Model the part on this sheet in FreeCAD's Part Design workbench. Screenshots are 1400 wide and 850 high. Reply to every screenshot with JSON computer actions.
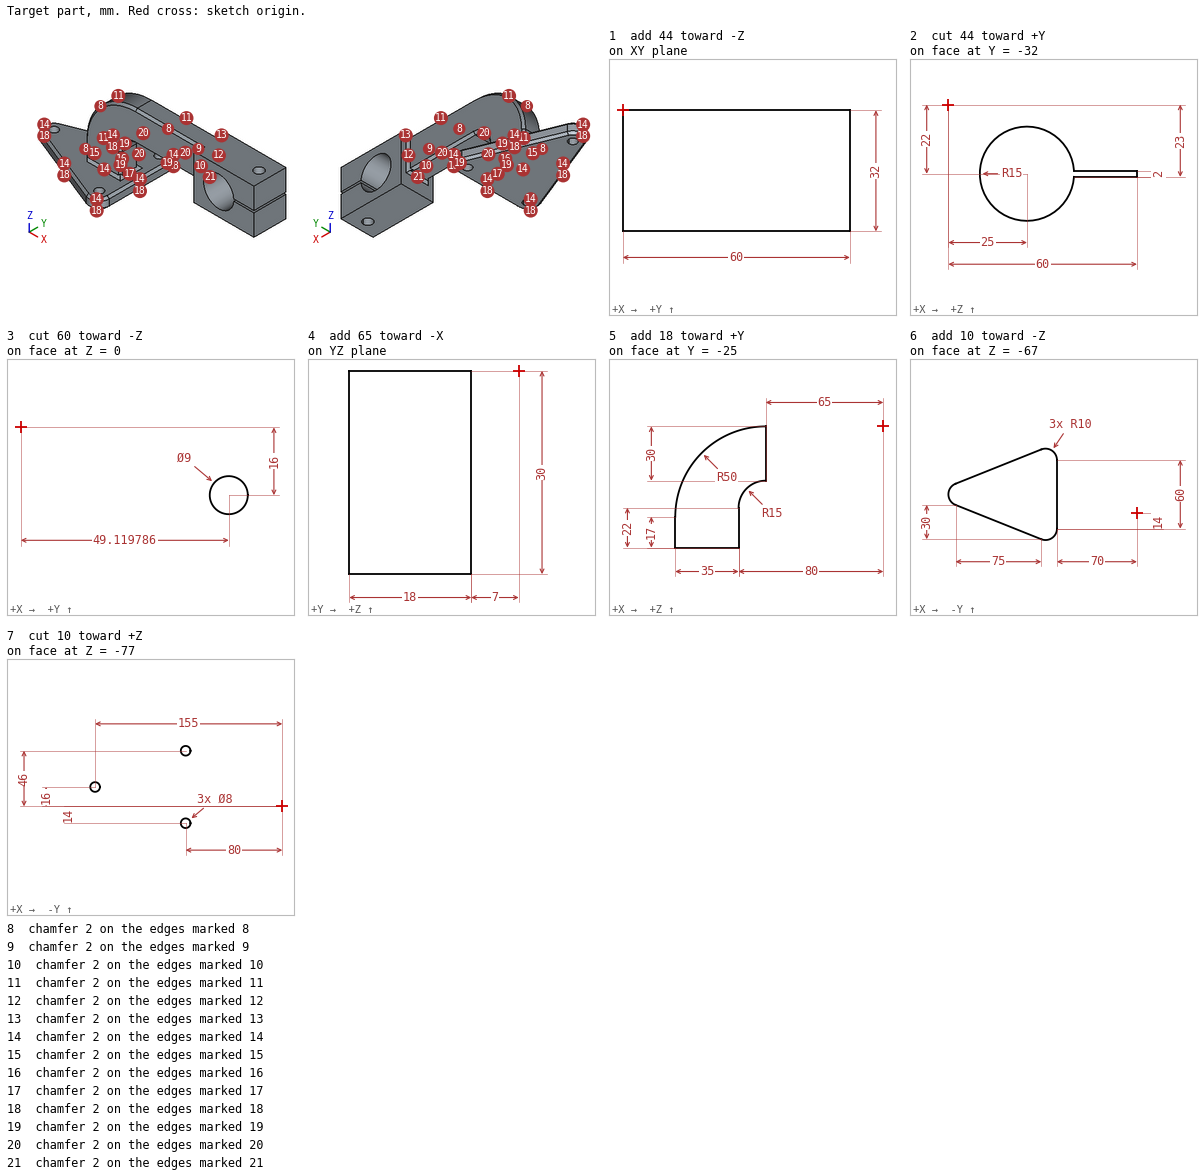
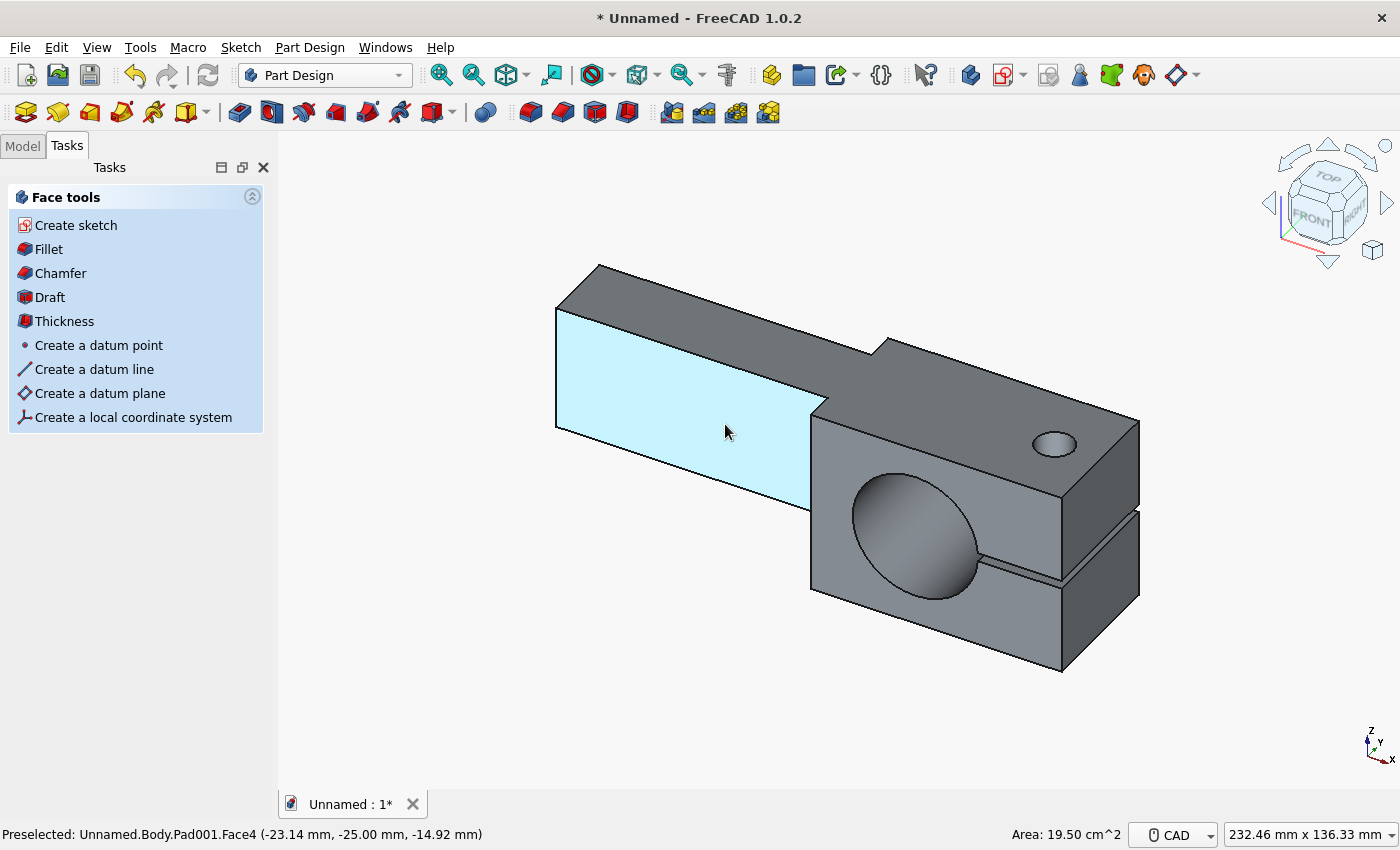
{"action": "left_click", "coordinate": [1004, 76]}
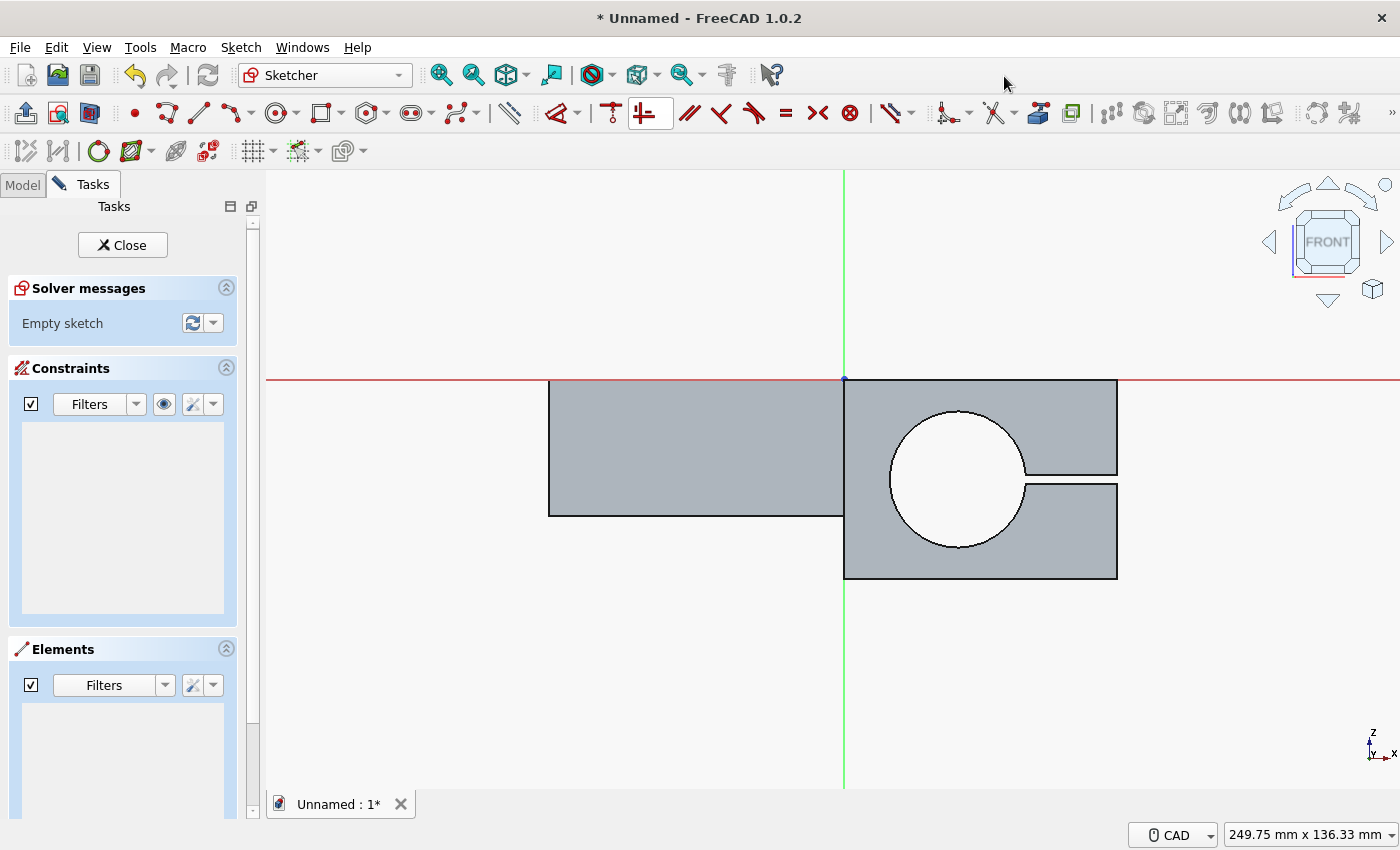
{"action": "left_click", "coordinate": [200, 114]}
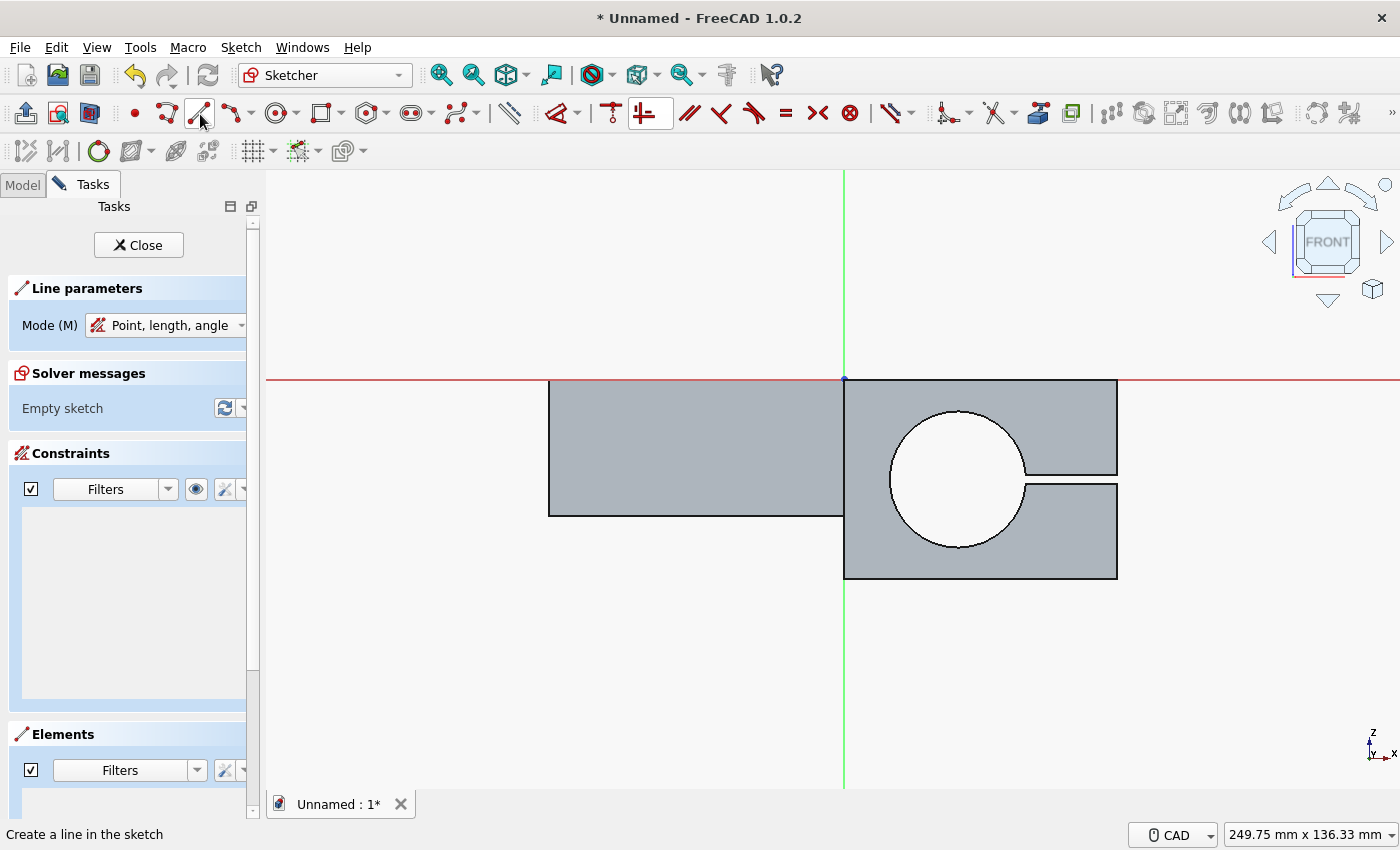
{"action": "left_click", "coordinate": [549, 516]}
{"action": "left_click", "coordinate": [549, 380]}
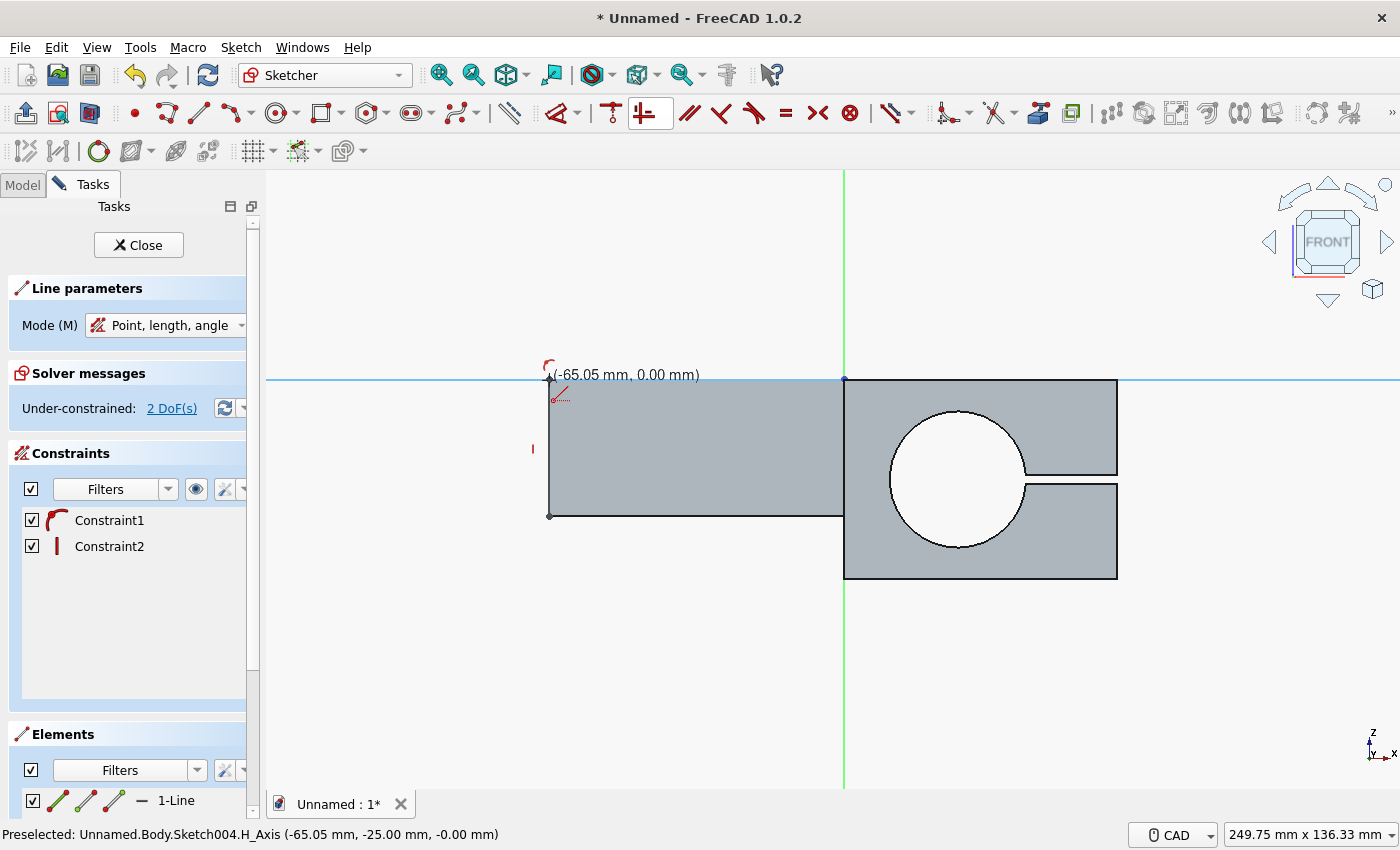
{"action": "left_click", "coordinate": [168, 114]}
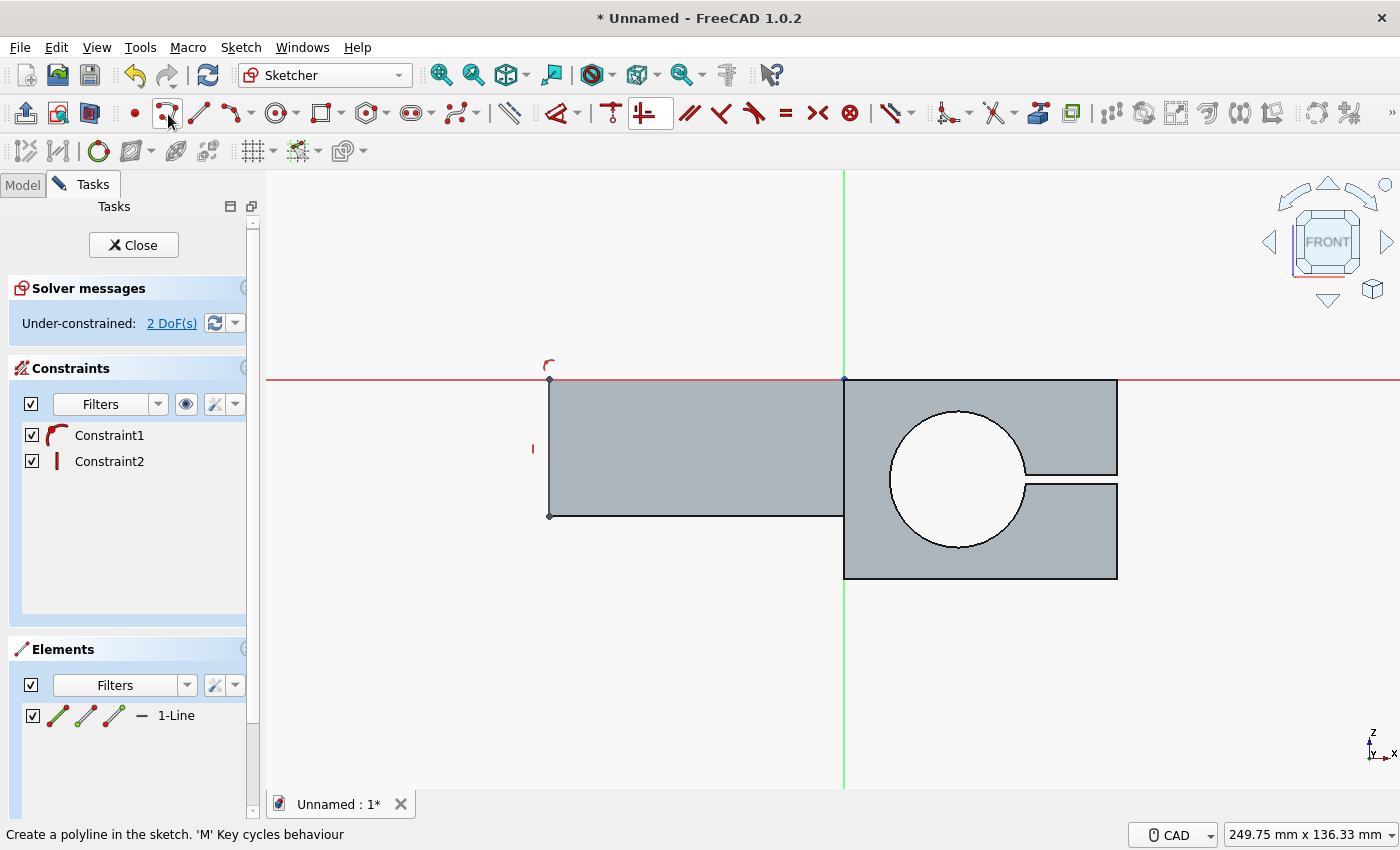
{"action": "left_click", "coordinate": [322, 607]}
{"action": "left_click", "coordinate": [322, 684]}
{"action": "left_click", "coordinate": [481, 684]}
{"action": "left_click", "coordinate": [481, 584]}
{"action": "right_click", "coordinate": [481, 584]}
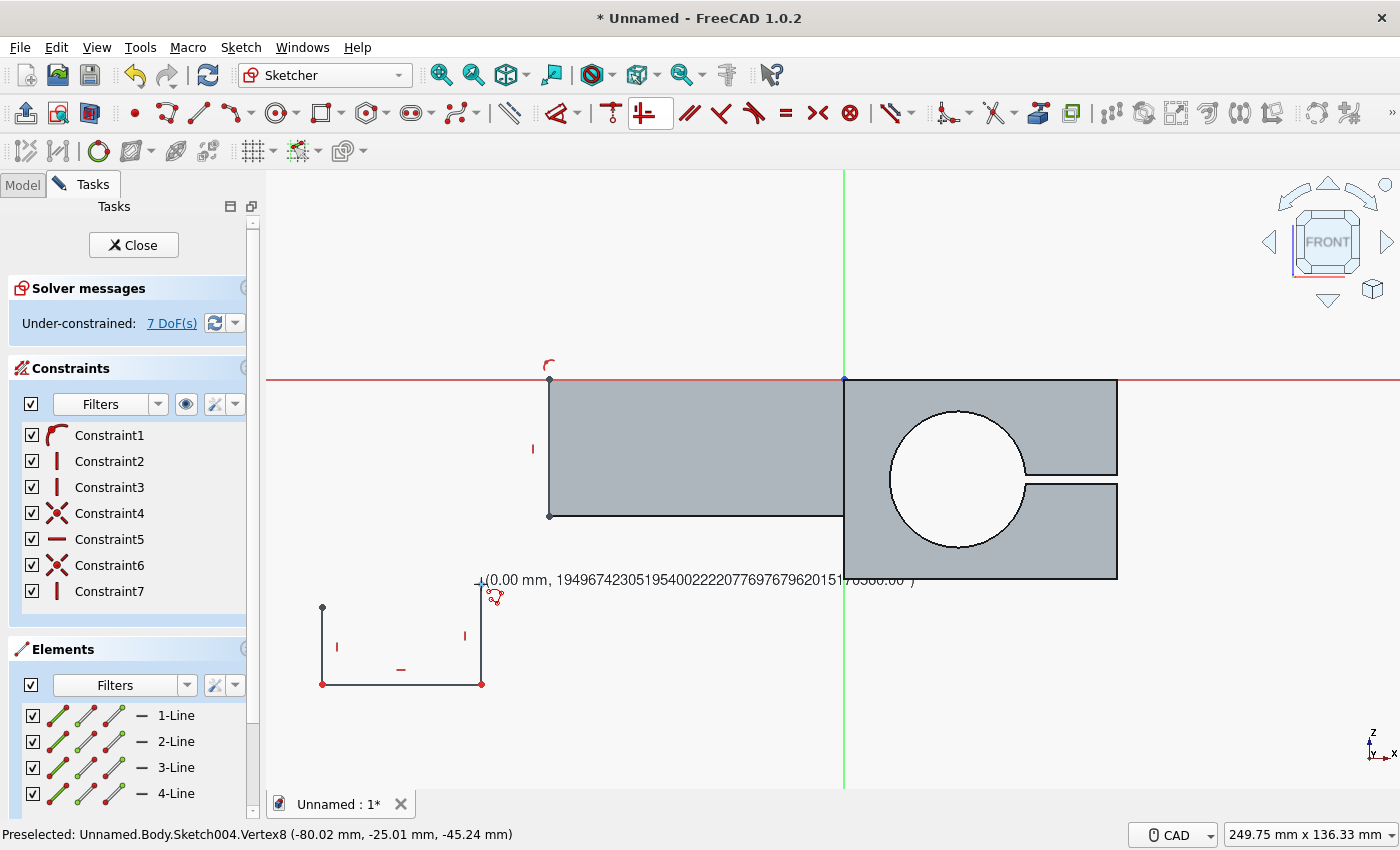
{"action": "key", "text": "g 3 a"}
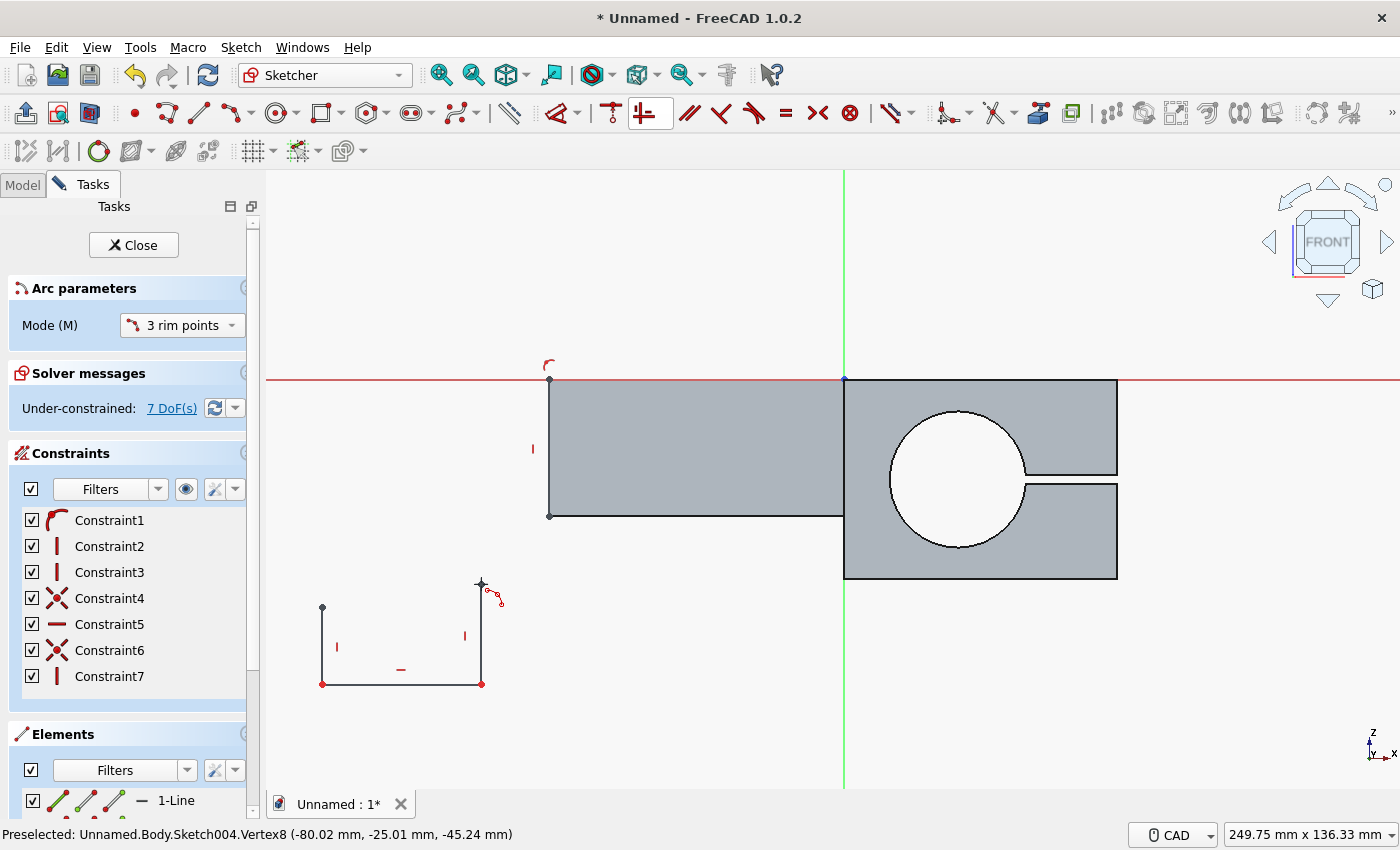
{"action": "left_click", "coordinate": [549, 380]}
{"action": "left_click", "coordinate": [322, 608]}
{"action": "left_click", "coordinate": [389, 446]}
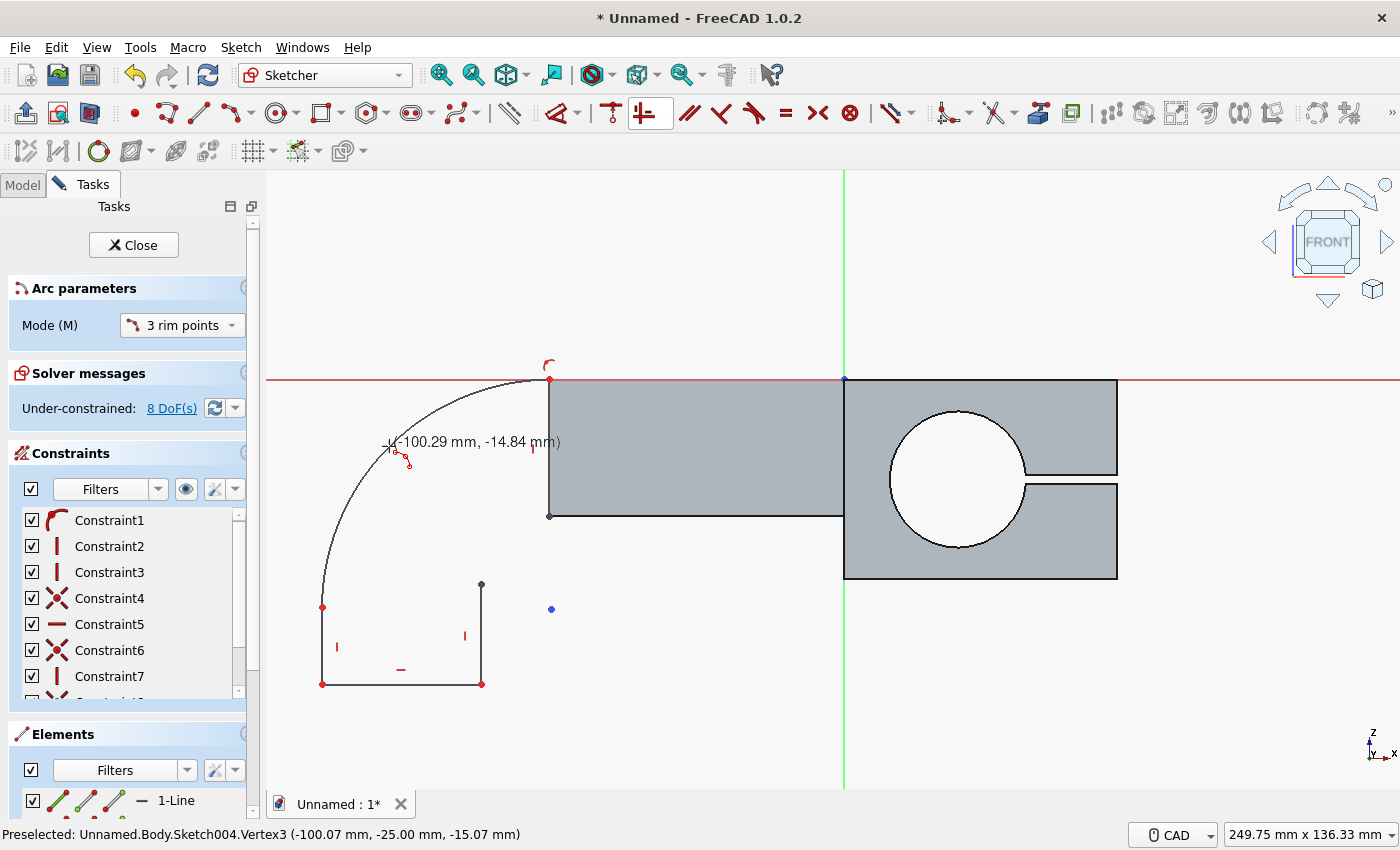
{"action": "left_click", "coordinate": [481, 585]}
{"action": "left_click", "coordinate": [549, 517]}
{"action": "left_click", "coordinate": [501, 536]}
{"action": "key", "text": "Escape"}